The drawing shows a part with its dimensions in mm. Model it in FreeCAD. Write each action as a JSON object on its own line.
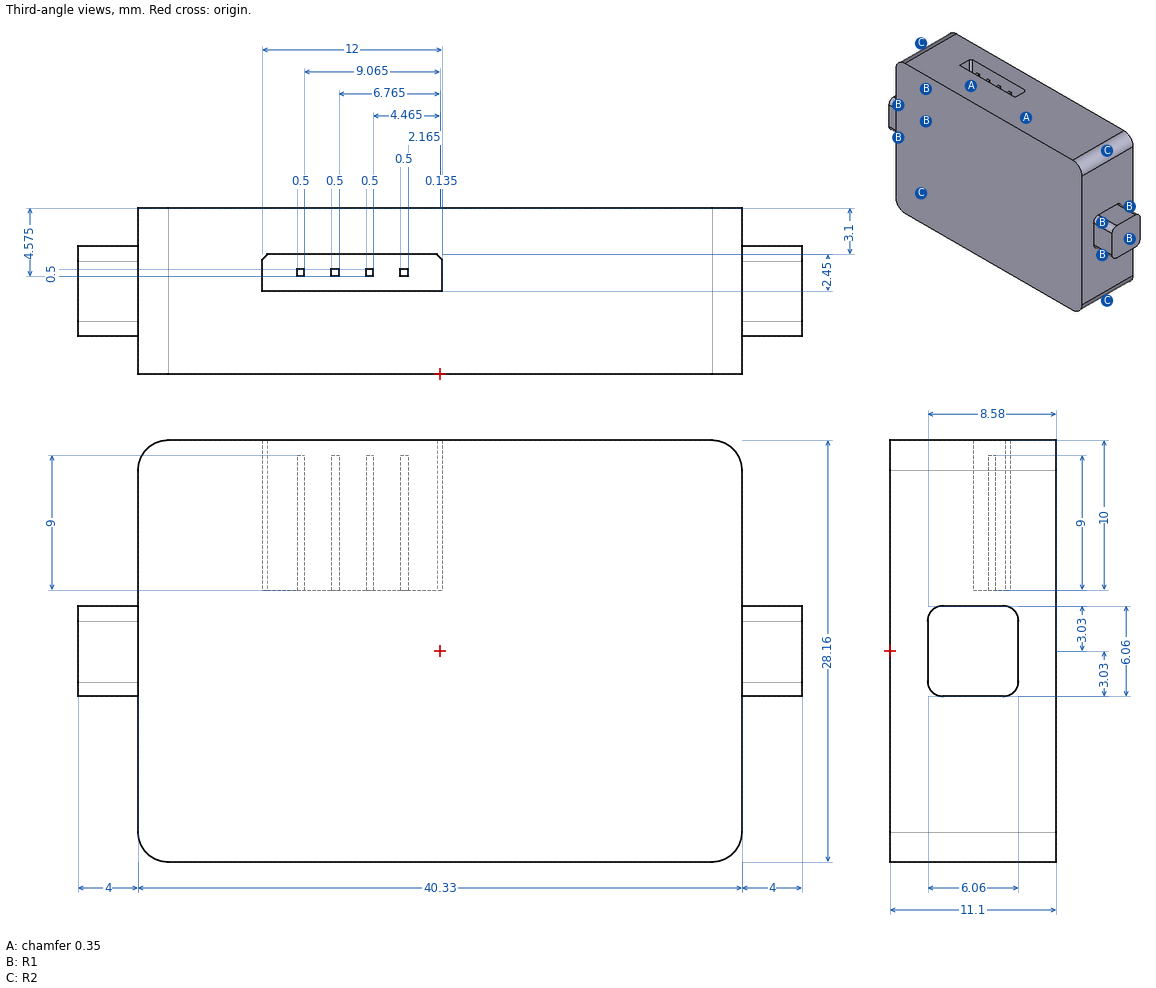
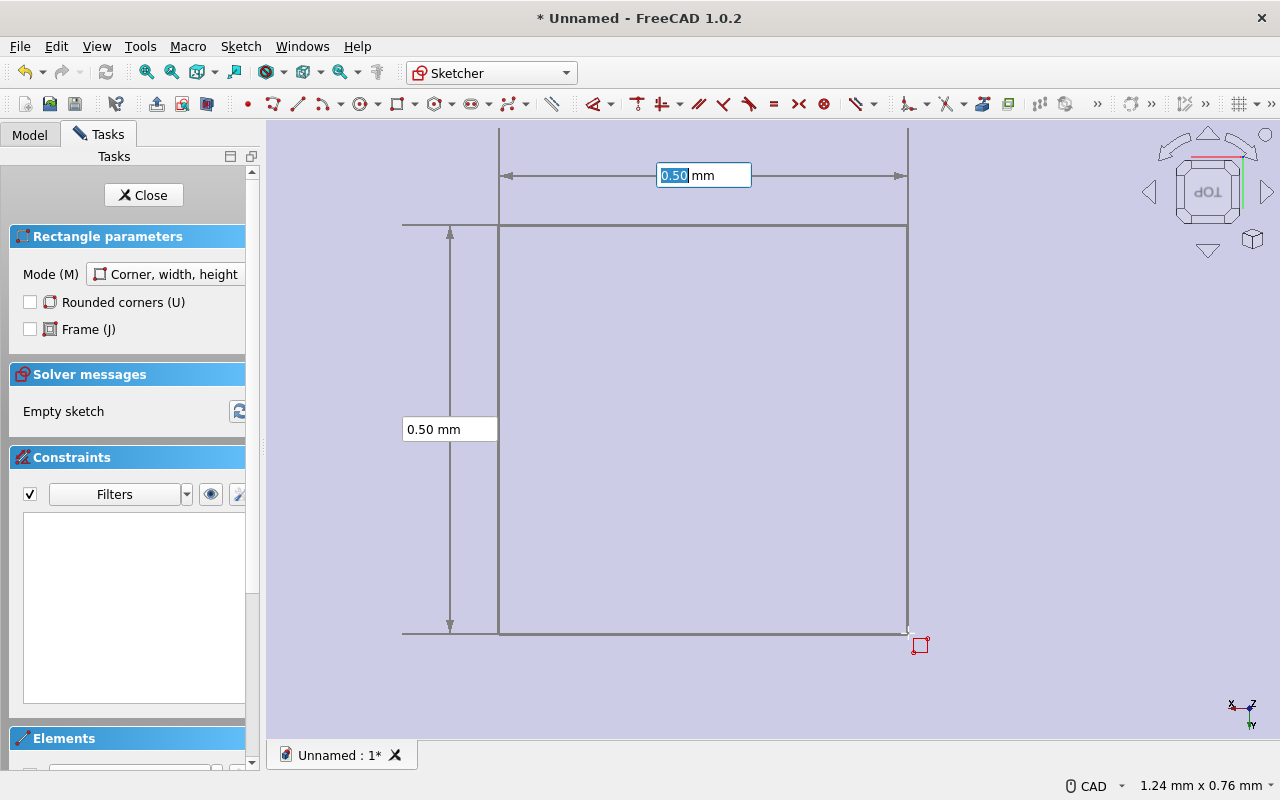
{"action": "type", "text": "0.5"}
{"action": "key", "text": "Tab"}
{"action": "type", "text": "0.5"}
{"action": "key", "text": "Return"}
{"action": "key", "text": "Escape"}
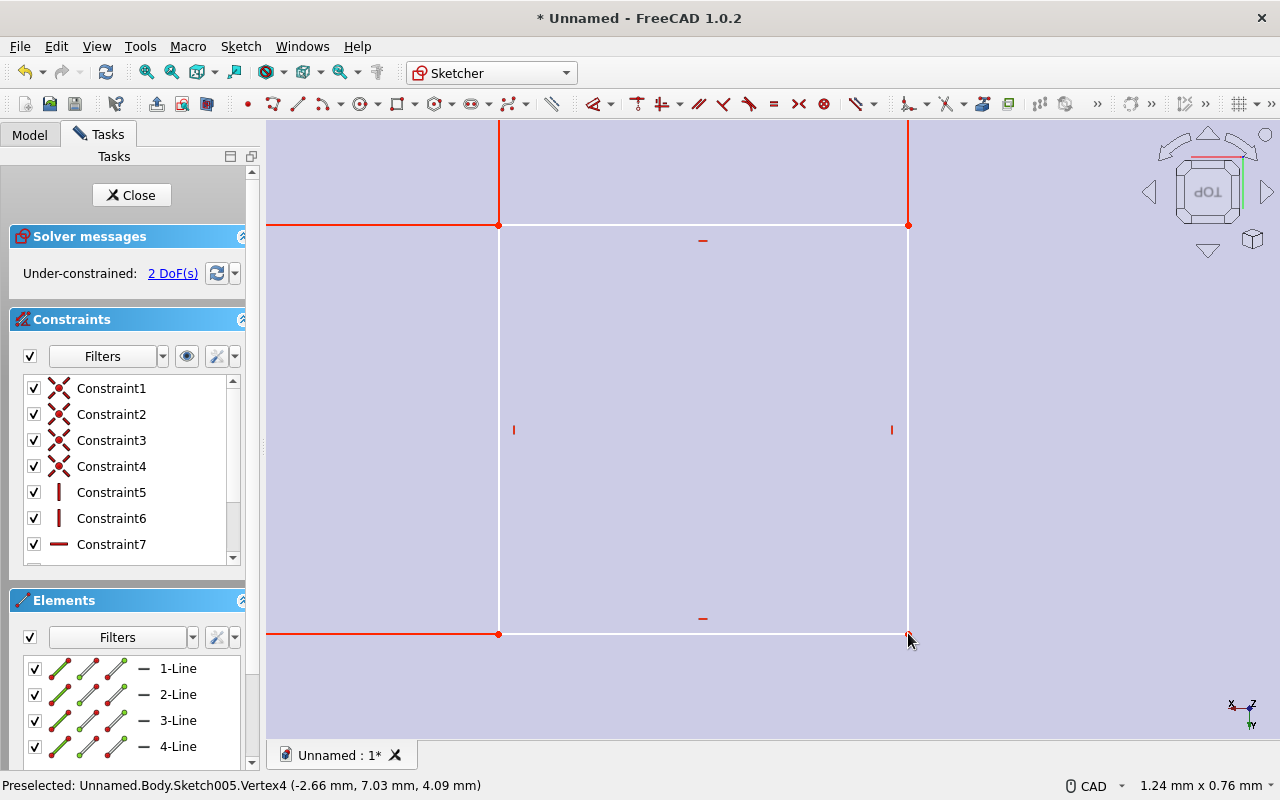
{"action": "left_click", "coordinate": [592, 104]}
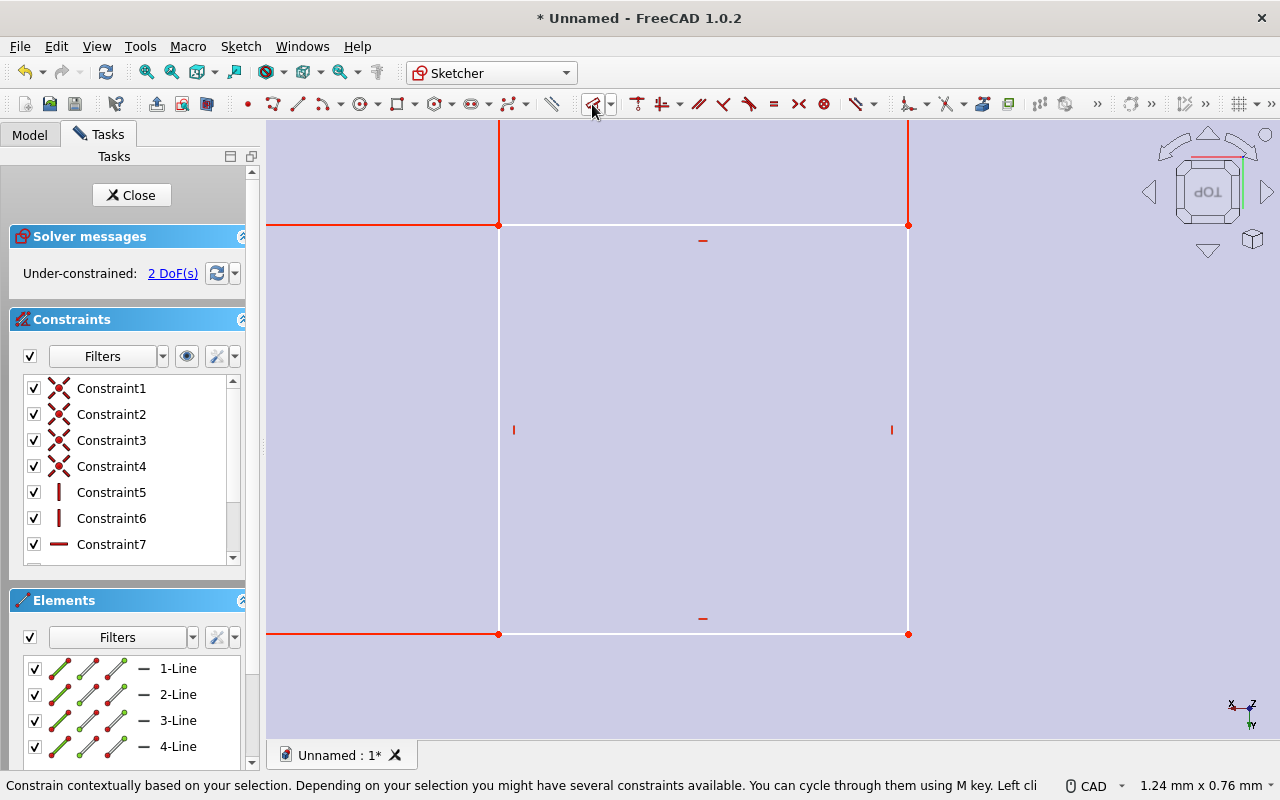
{"action": "left_click", "coordinate": [499, 225]}
{"action": "left_click", "coordinate": [396, 191]}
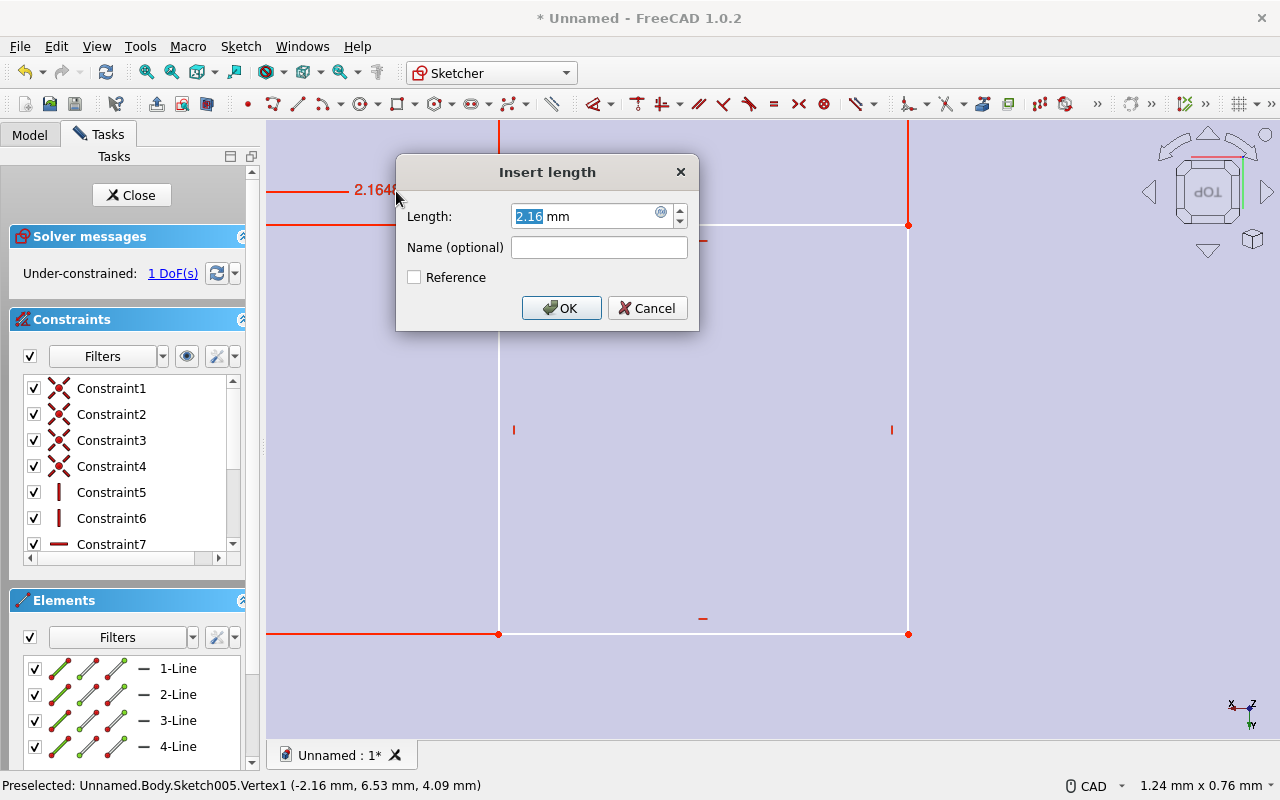
{"action": "type", "text": "2.165"}
{"action": "key", "text": "Return"}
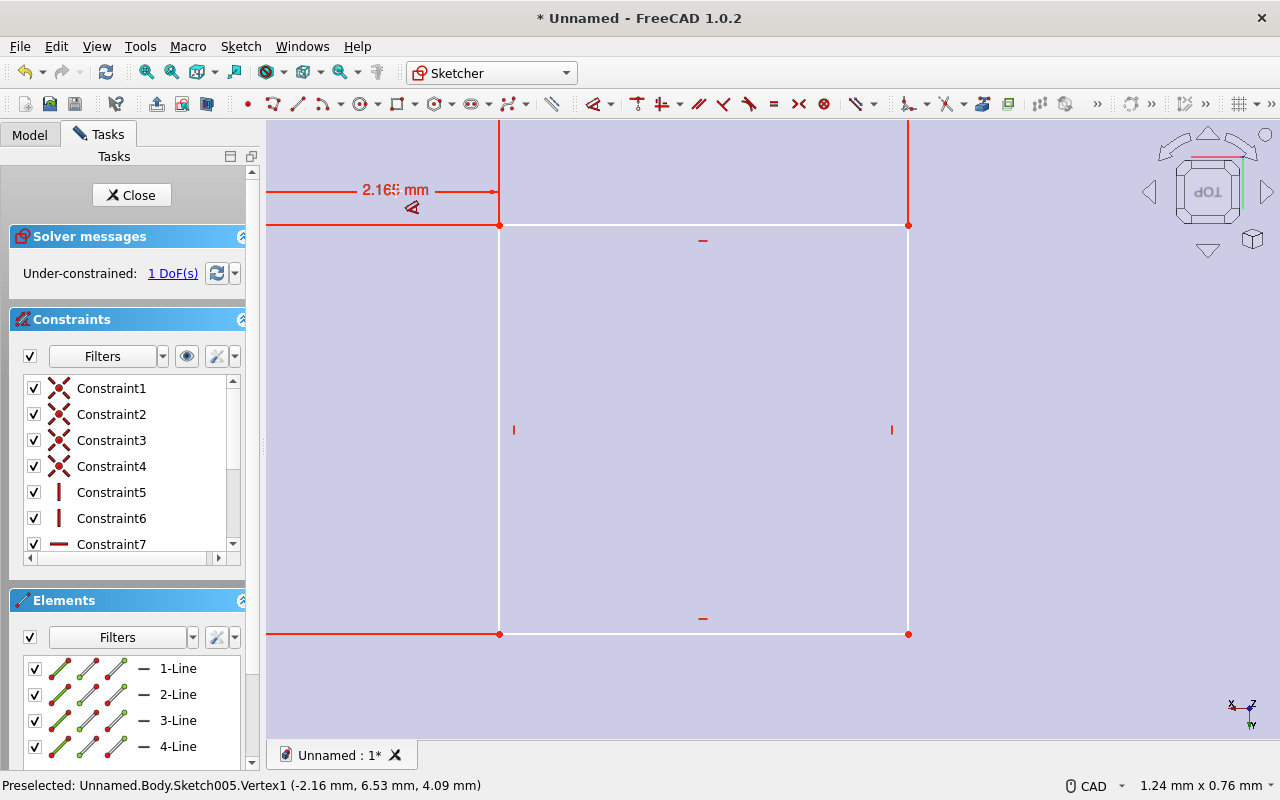
{"action": "left_click", "coordinate": [499, 225]}
{"action": "left_click", "coordinate": [533, 468]}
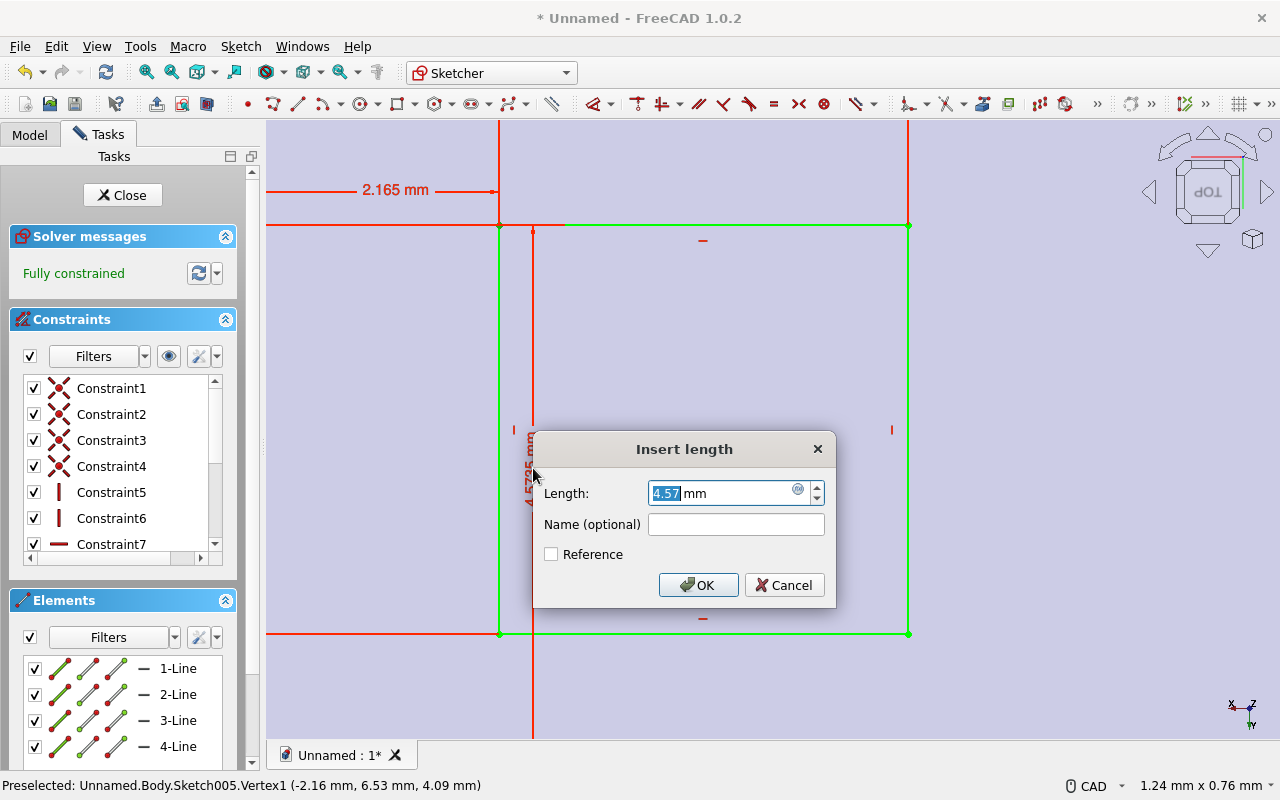
{"action": "type", "text": "4.575"}
{"action": "key", "text": "Return"}
{"action": "key", "text": "Escape"}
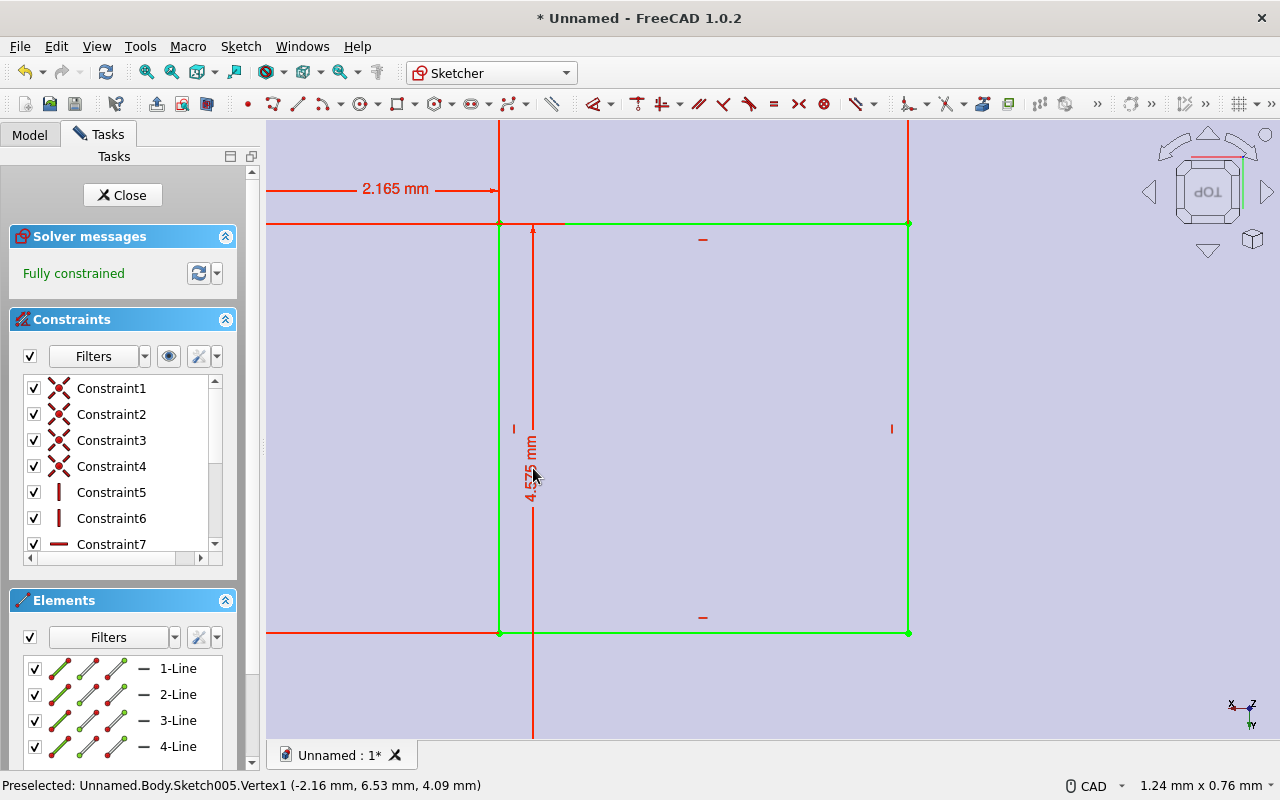
{"action": "left_click", "coordinate": [123, 195]}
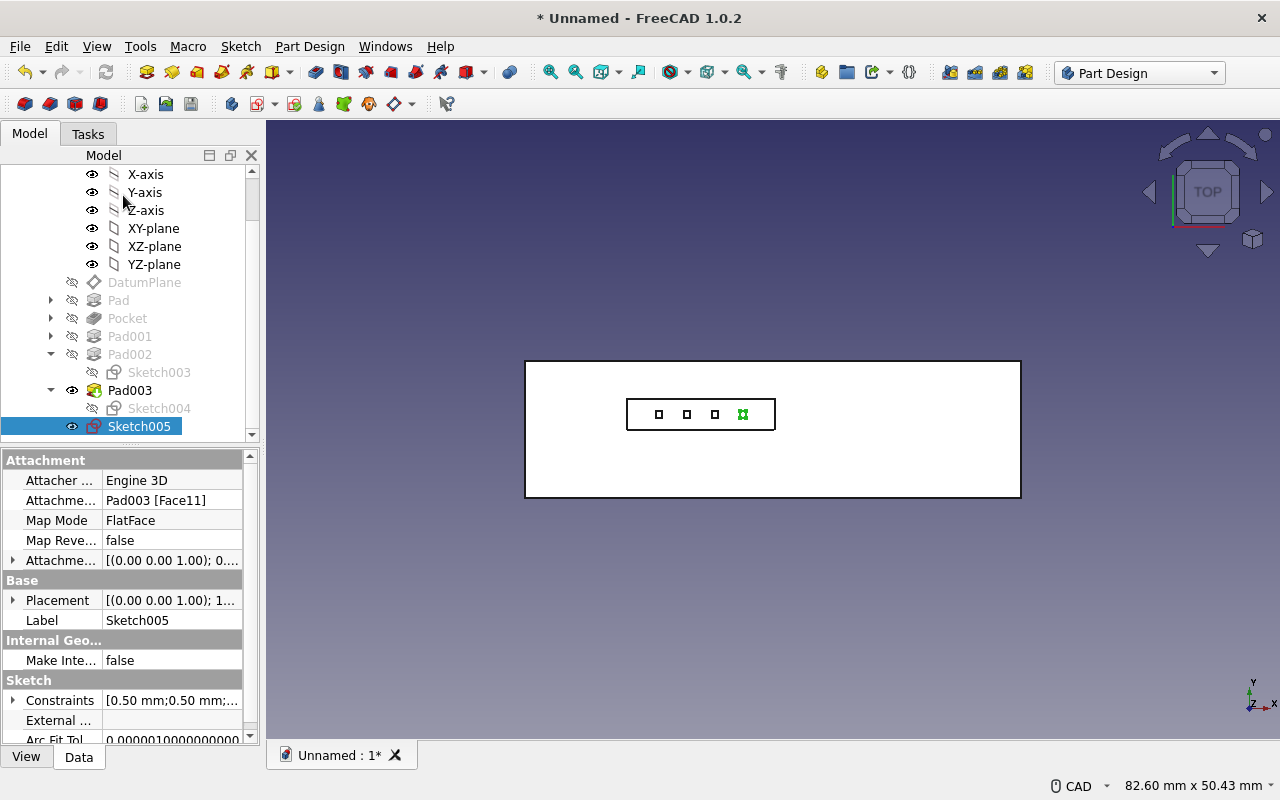
{"action": "left_click", "coordinate": [147, 72]}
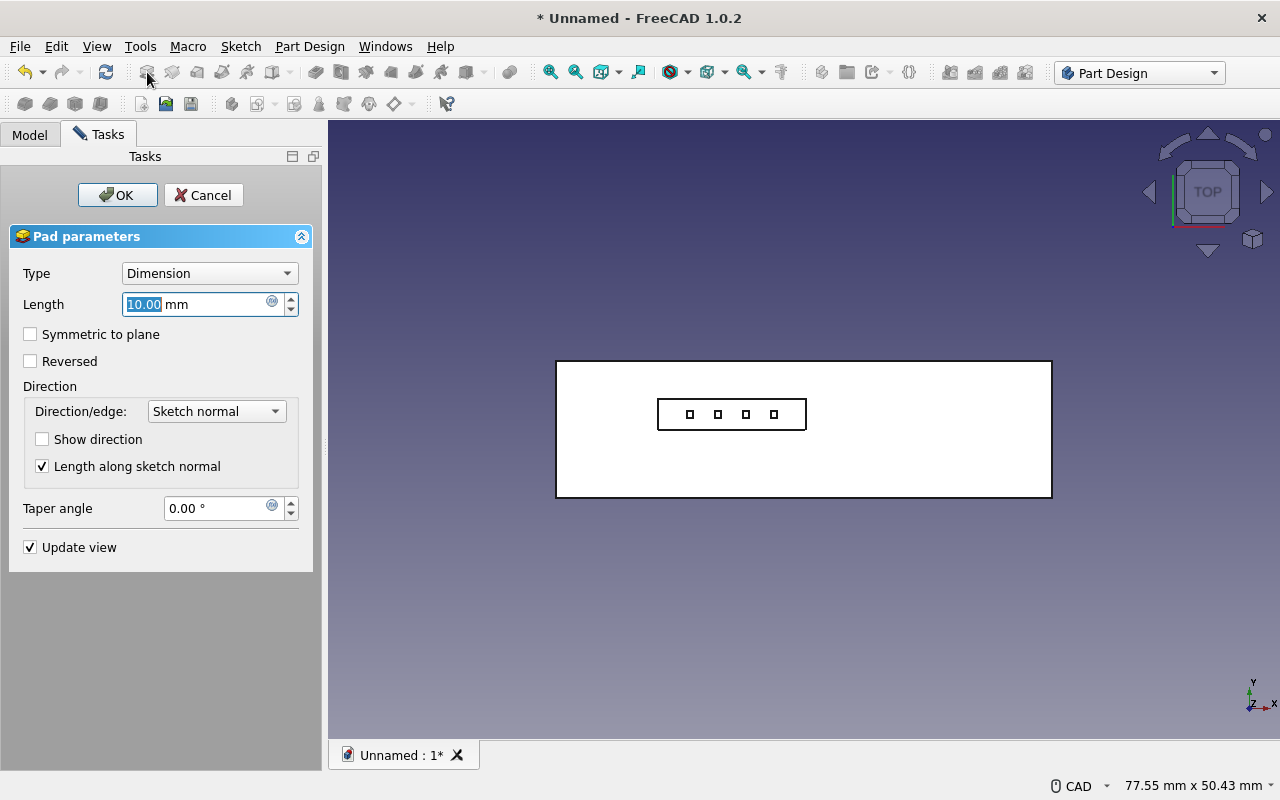
{"action": "type", "text": "9"}
{"action": "key", "text": "Tab"}